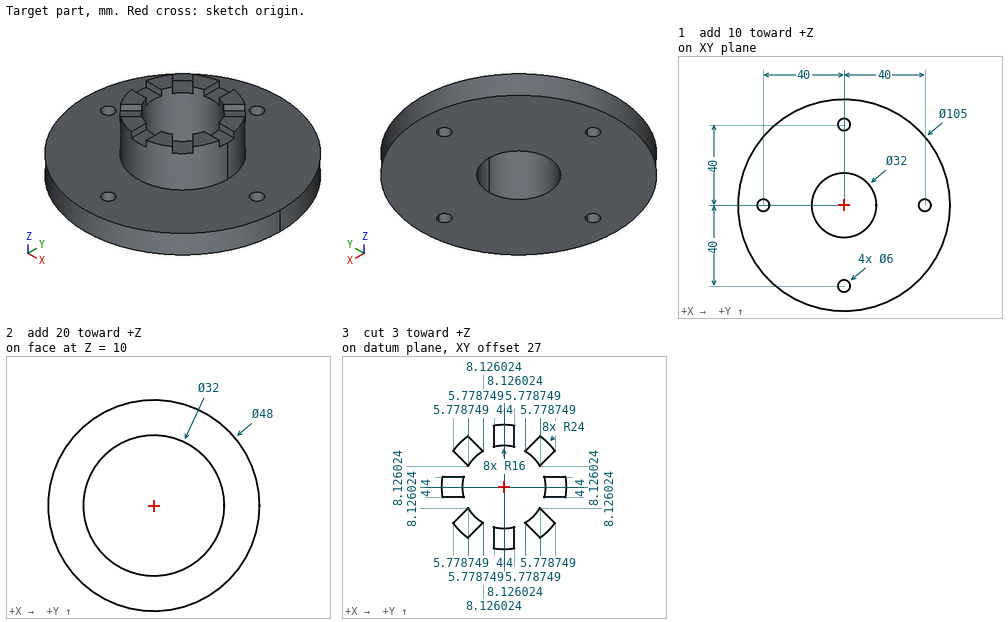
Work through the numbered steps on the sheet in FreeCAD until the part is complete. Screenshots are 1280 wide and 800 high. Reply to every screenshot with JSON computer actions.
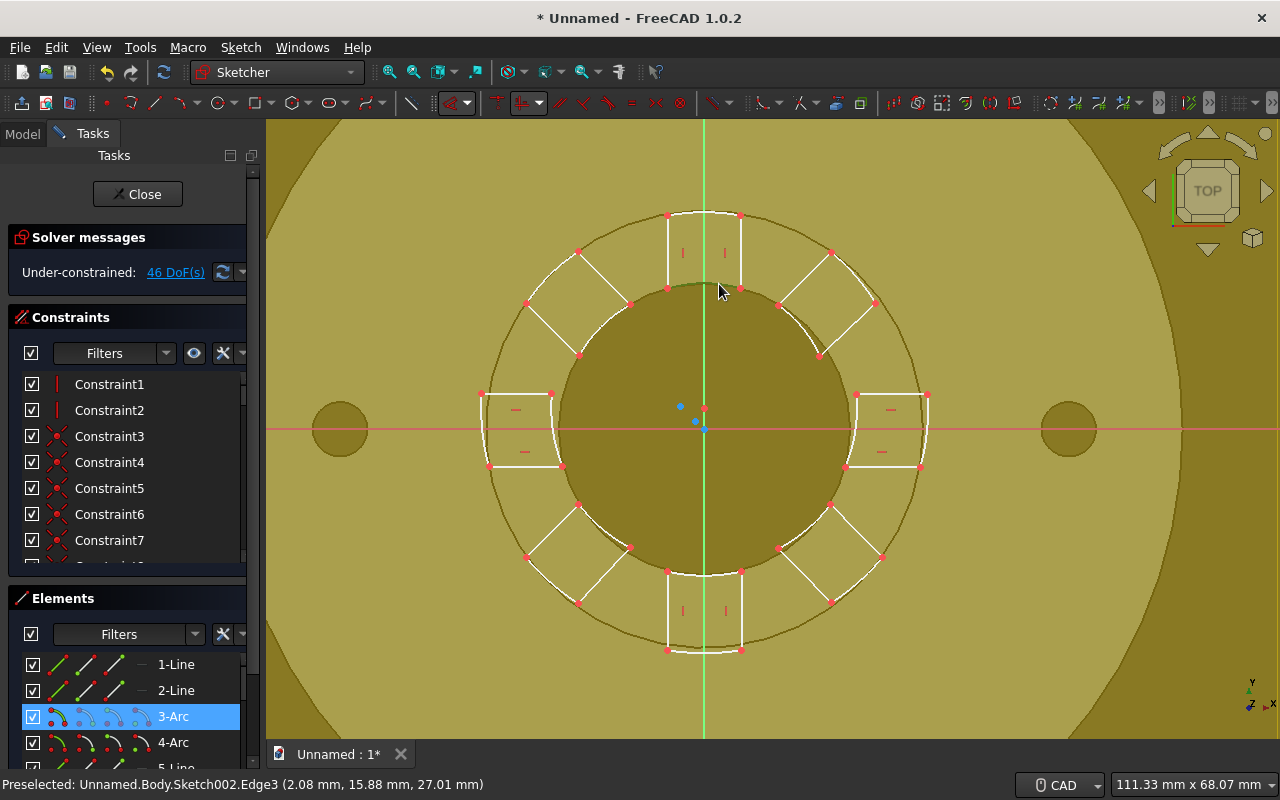
{"action": "left_click", "coordinate": [612, 317]}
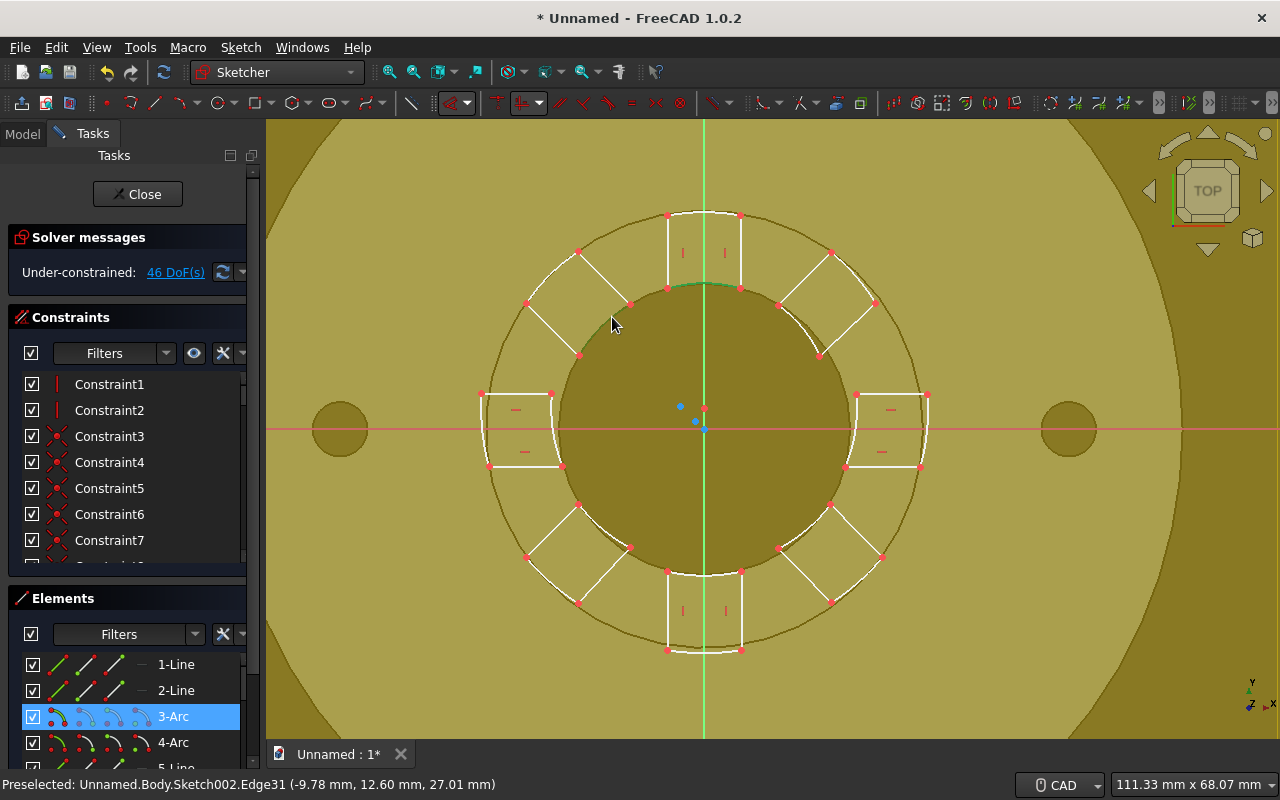
{"action": "left_click", "coordinate": [498, 104]}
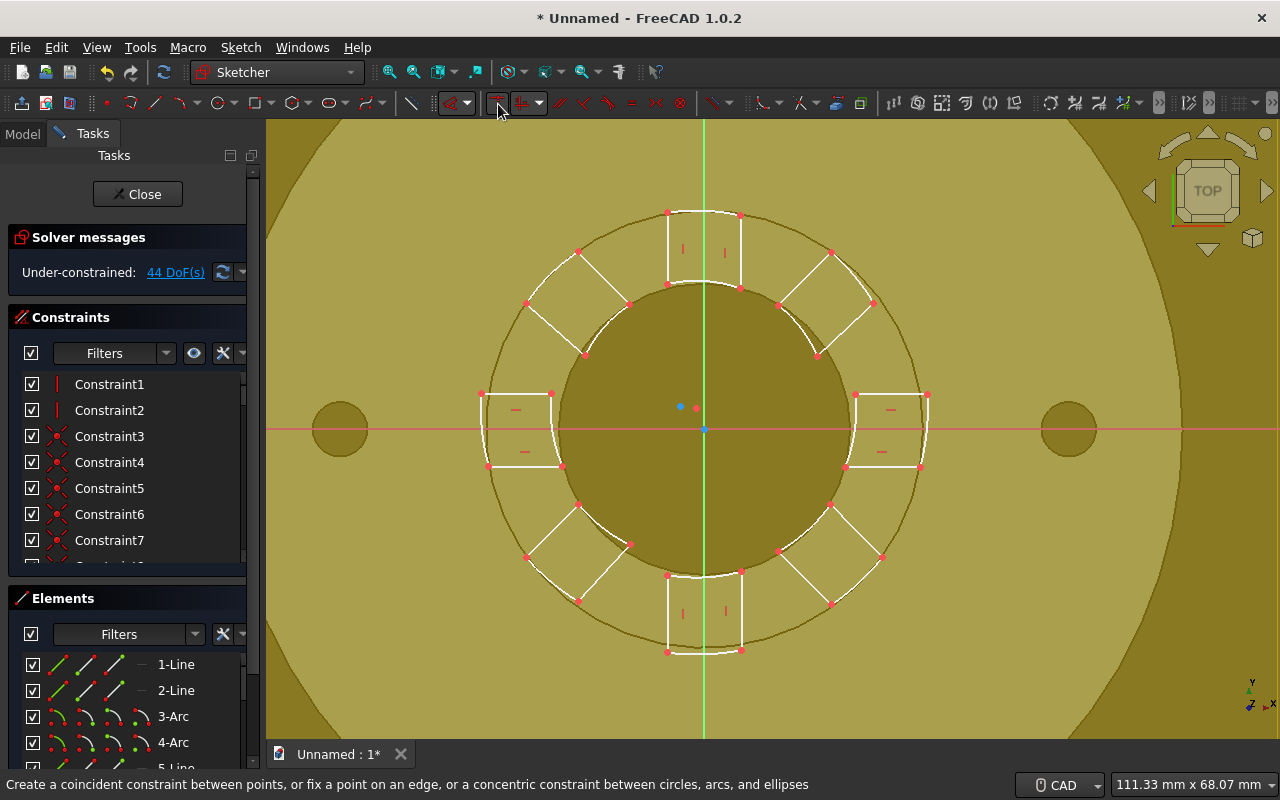
{"action": "left_click", "coordinate": [719, 283]}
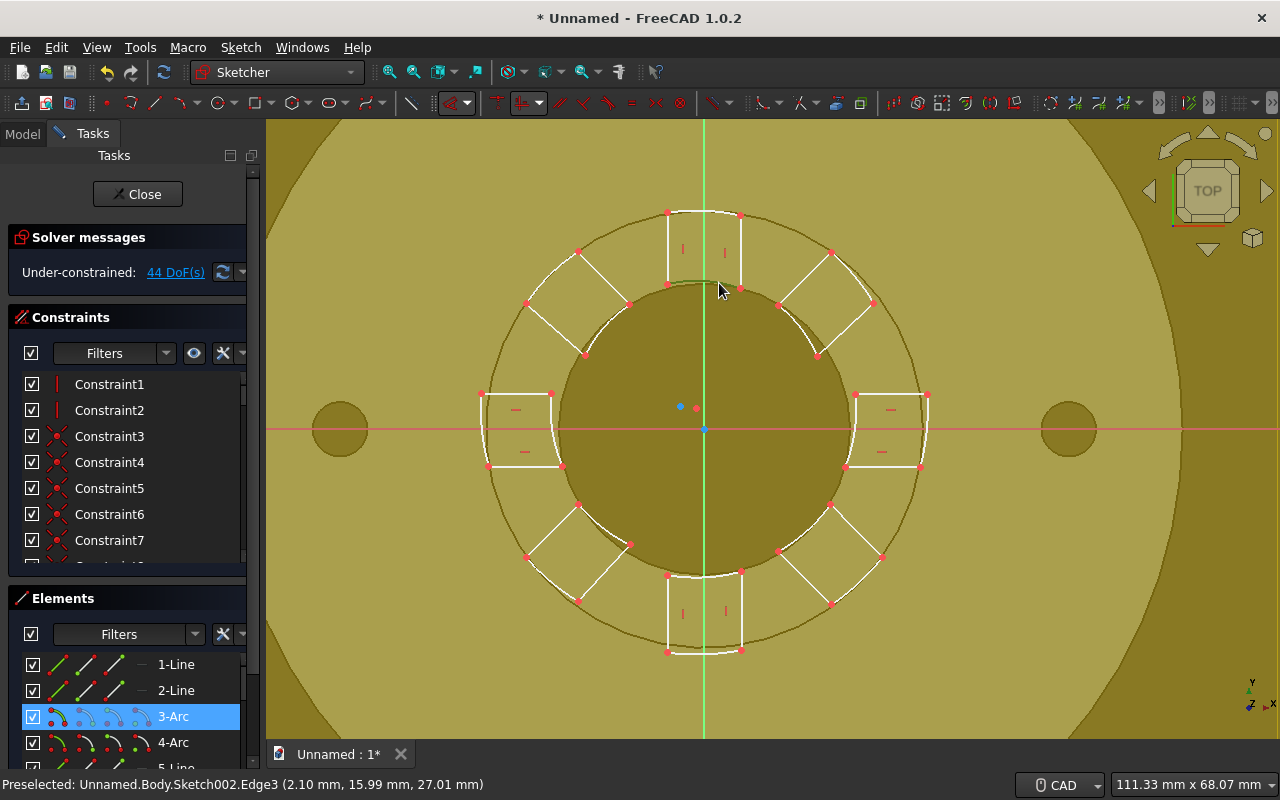
{"action": "left_click", "coordinate": [560, 265]}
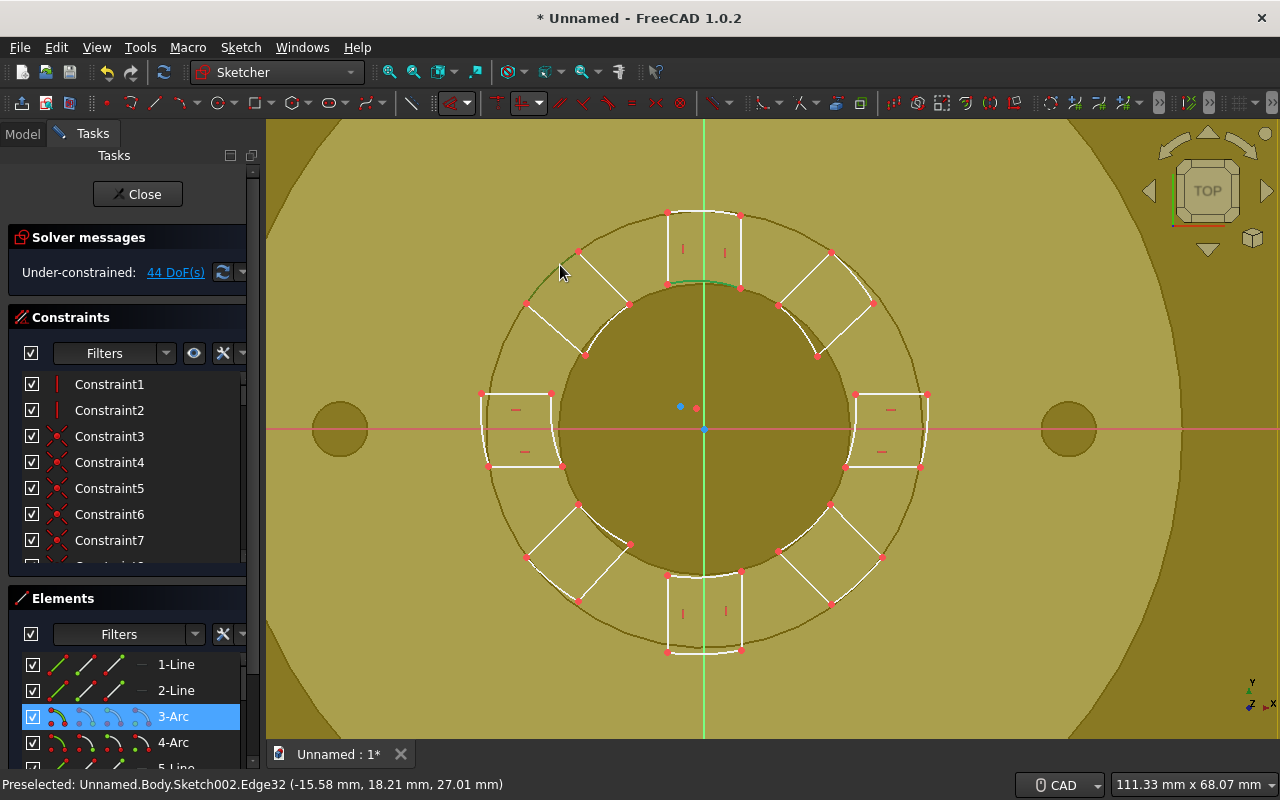
{"action": "left_click", "coordinate": [498, 104]}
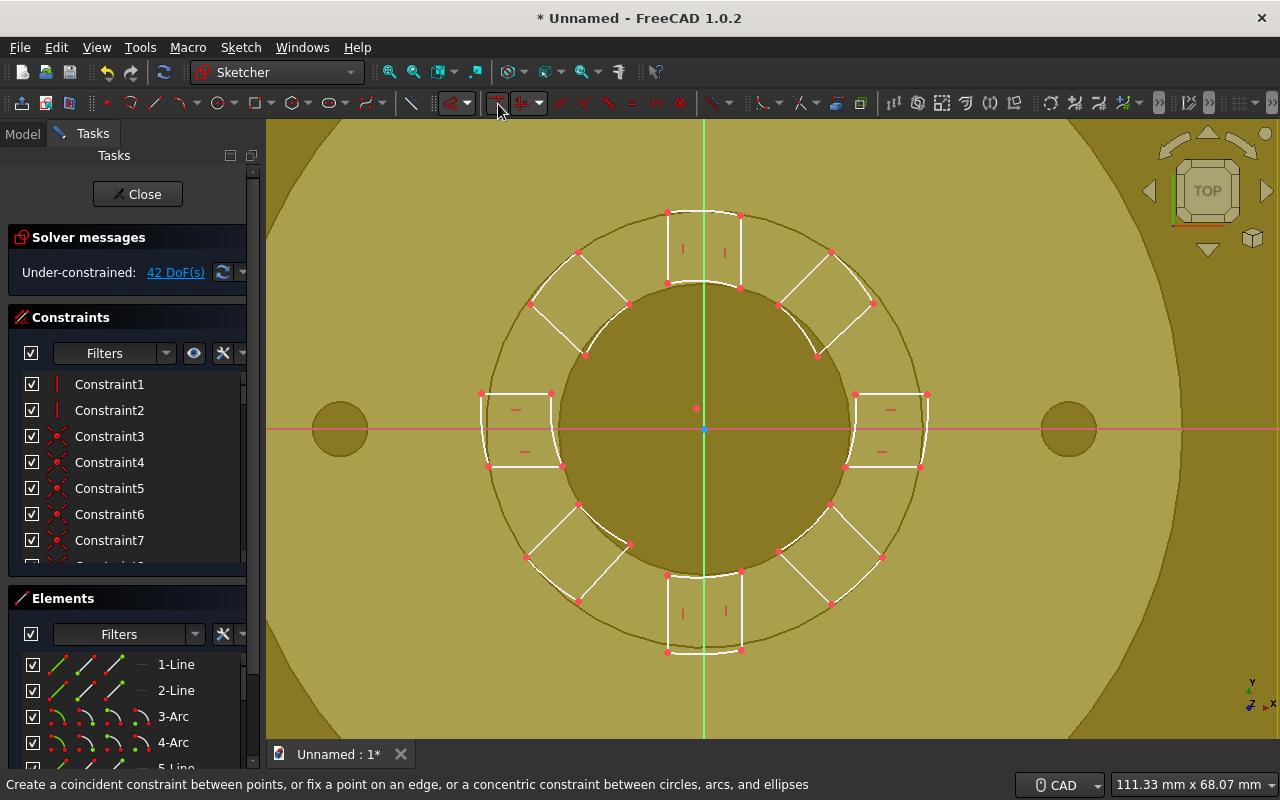
{"action": "left_click_drag", "start_coordinate": [686, 398], "coordinate": [714, 439]}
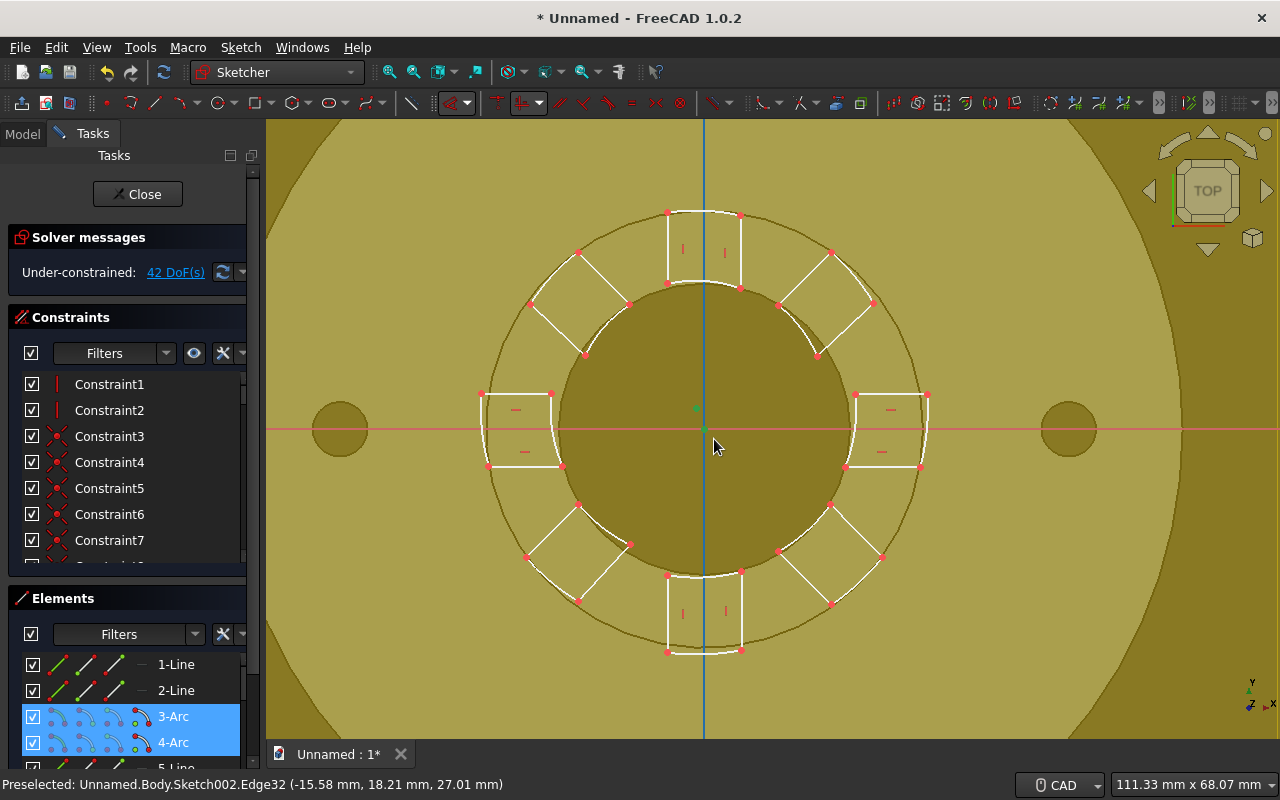
{"action": "left_click", "coordinate": [498, 104]}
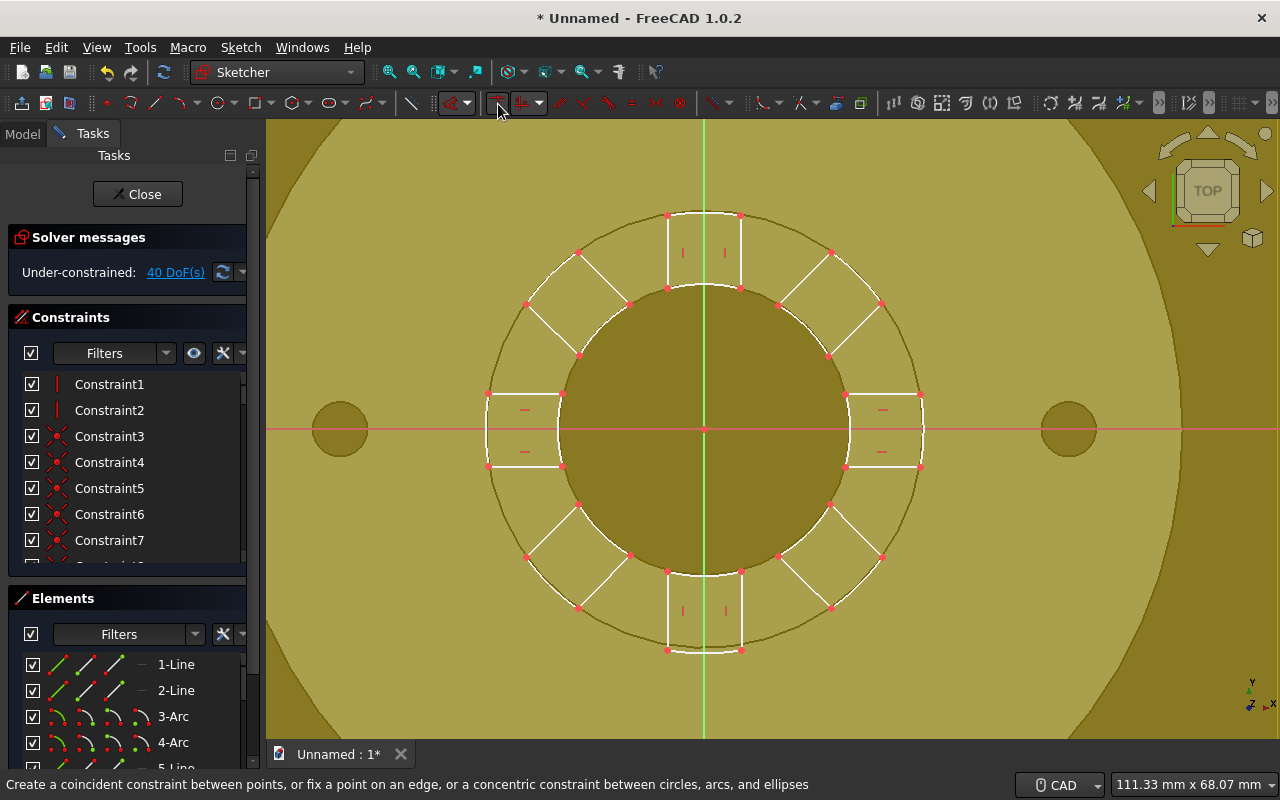
{"action": "left_click", "coordinate": [719, 285]}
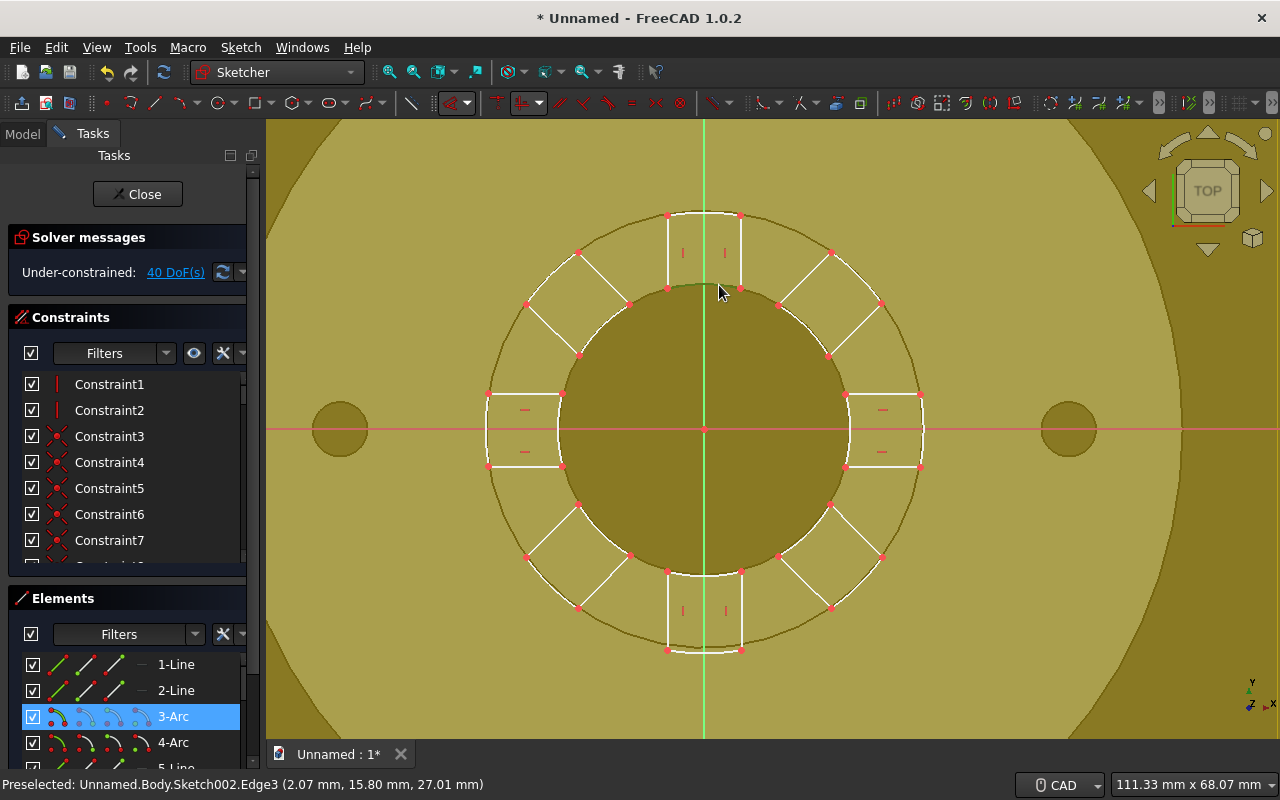
{"action": "left_click", "coordinate": [816, 338]}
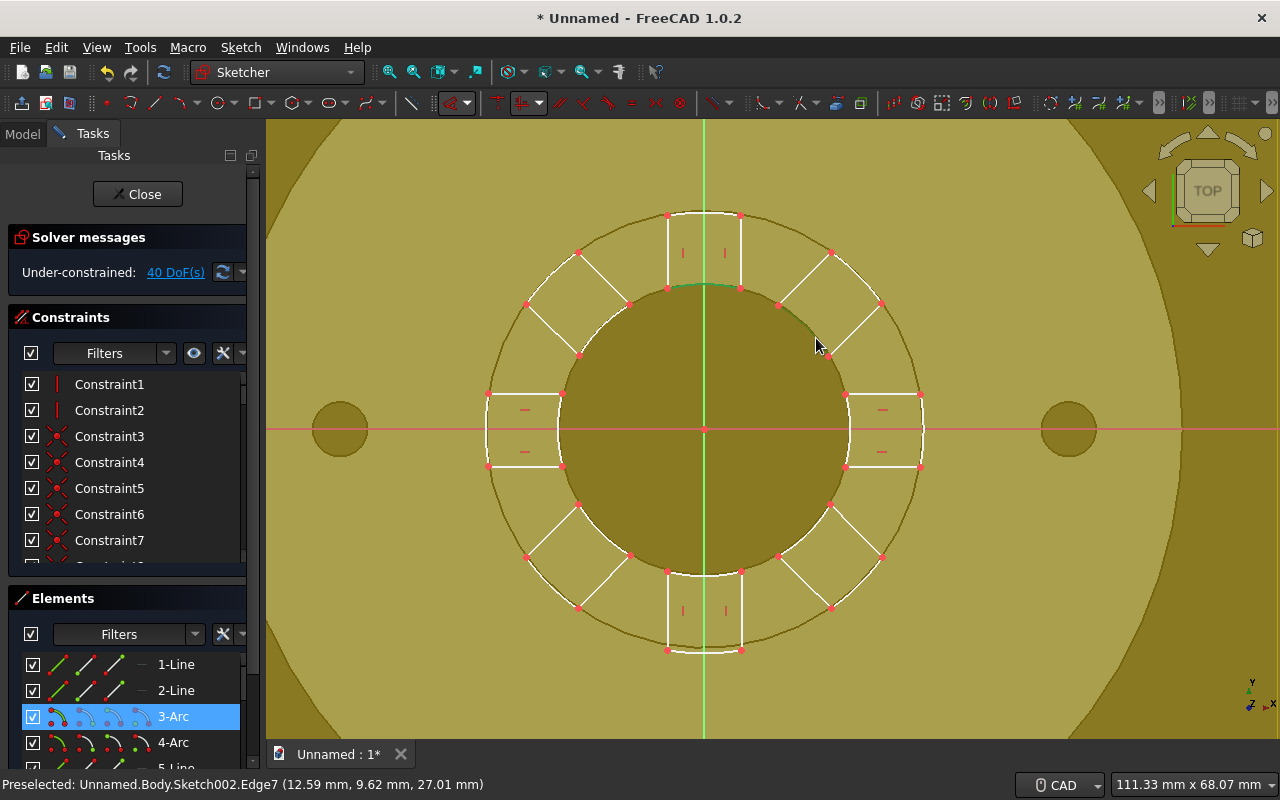
{"action": "left_click", "coordinate": [849, 445]}